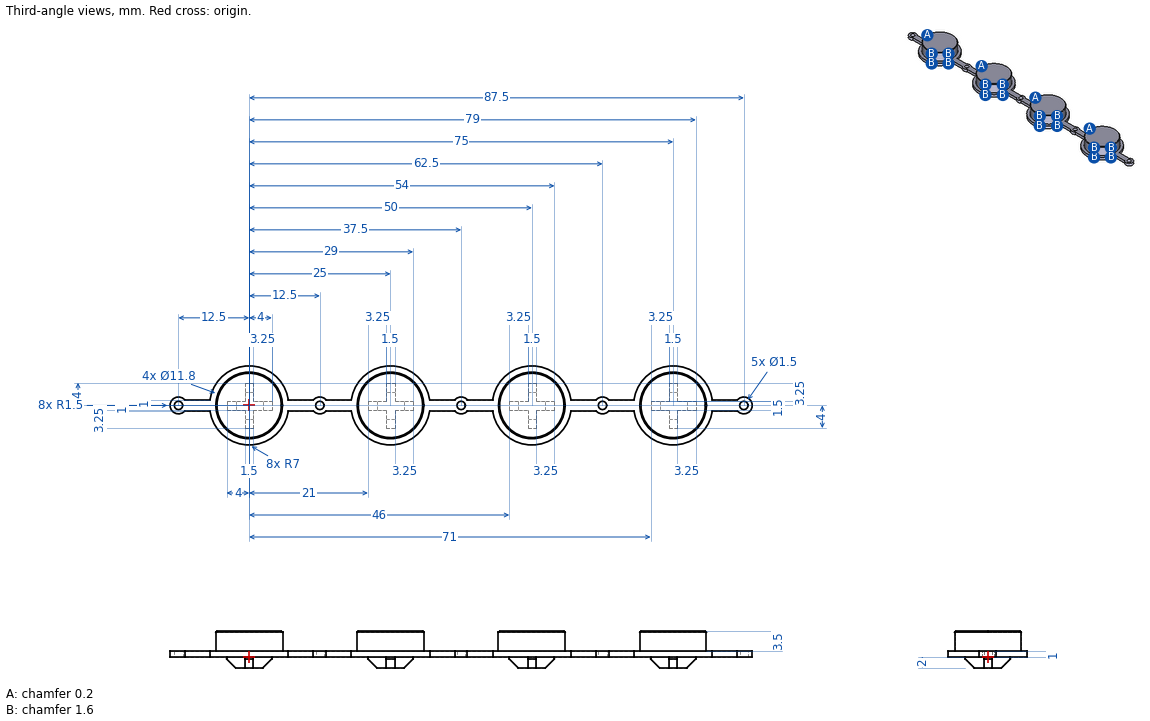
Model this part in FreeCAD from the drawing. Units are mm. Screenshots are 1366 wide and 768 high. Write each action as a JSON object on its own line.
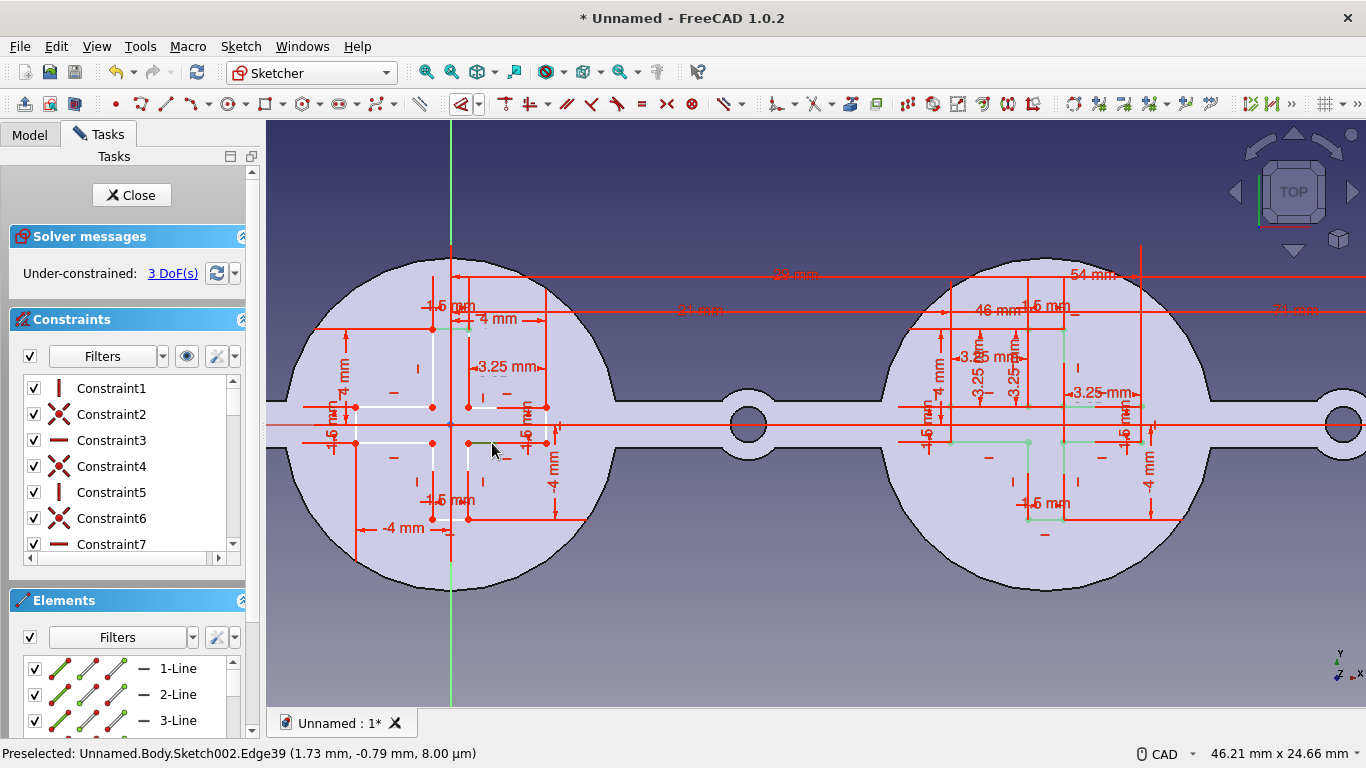
{"action": "key", "text": "l"}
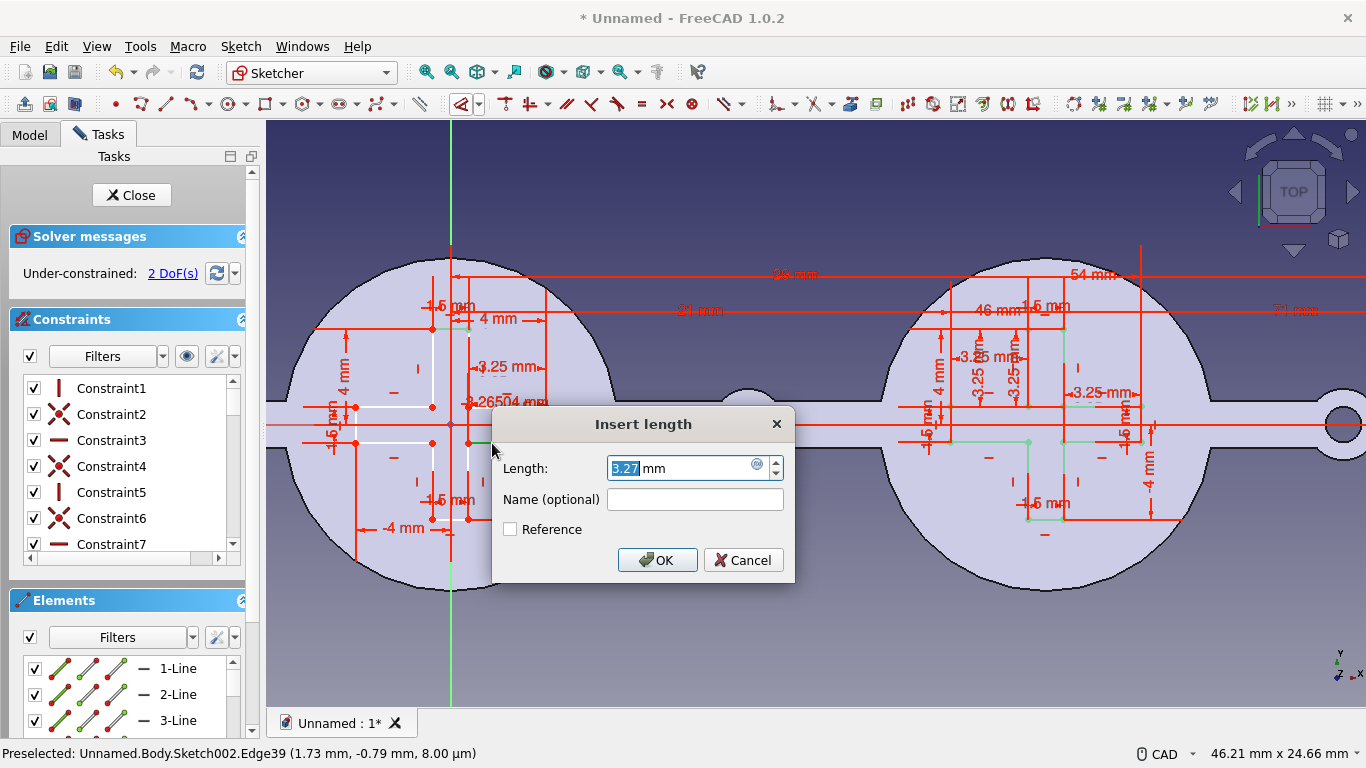
{"action": "type", "text": "3.25"}
{"action": "key", "text": "Return"}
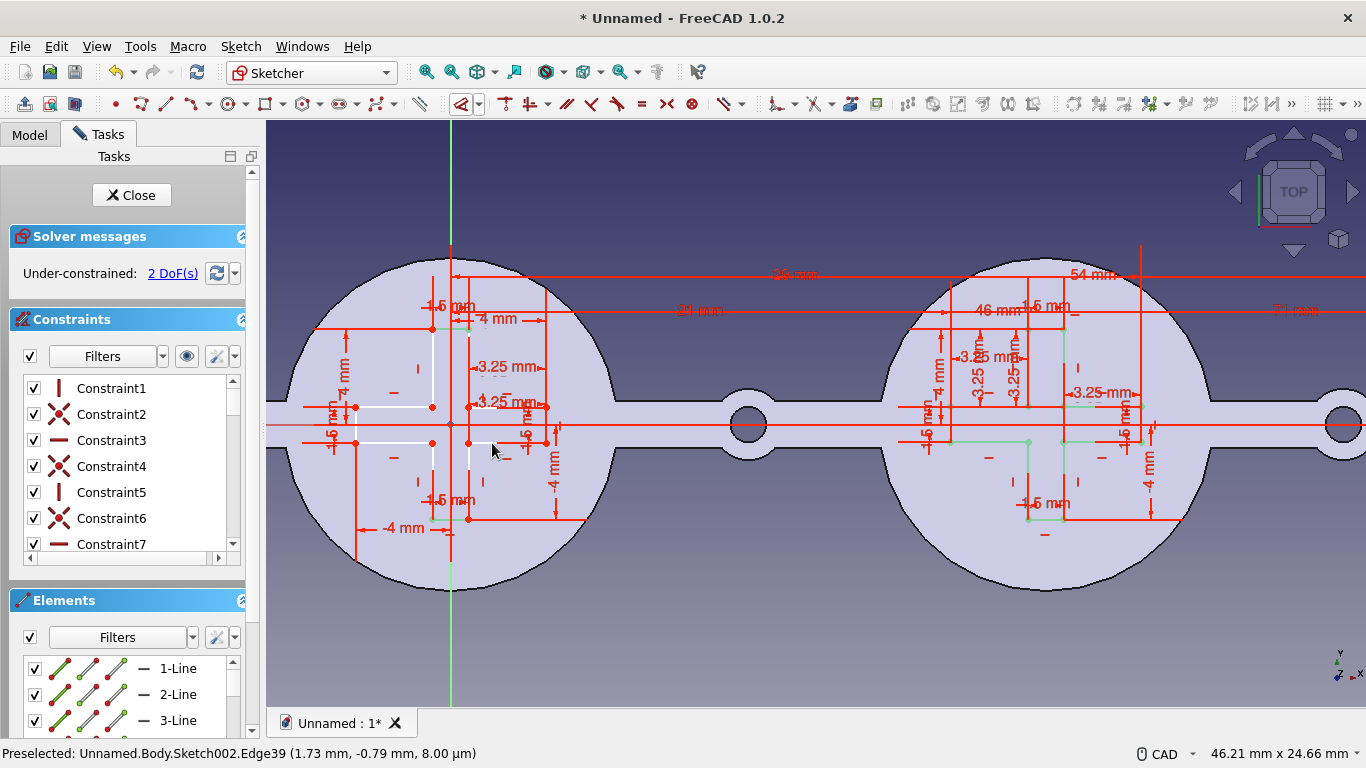
{"action": "left_click", "coordinate": [469, 466]}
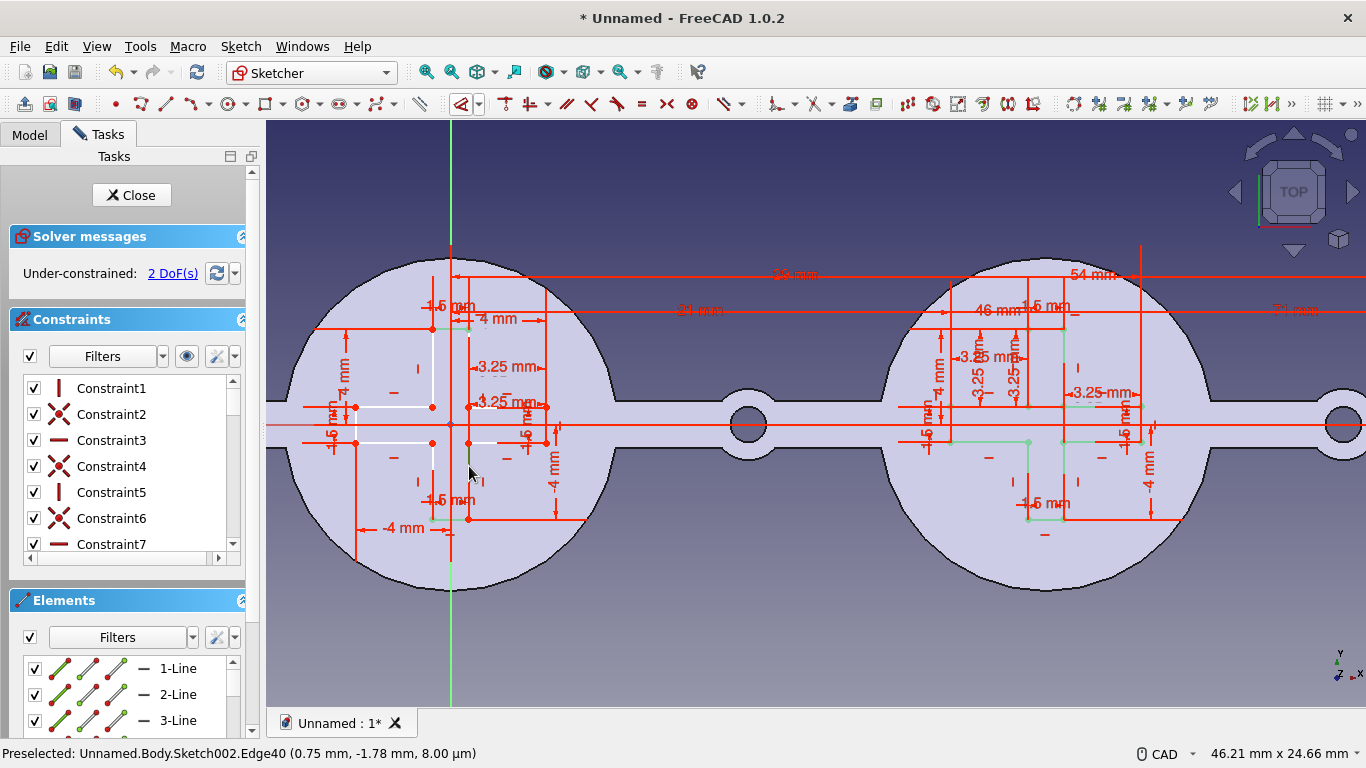
{"action": "key", "text": "i"}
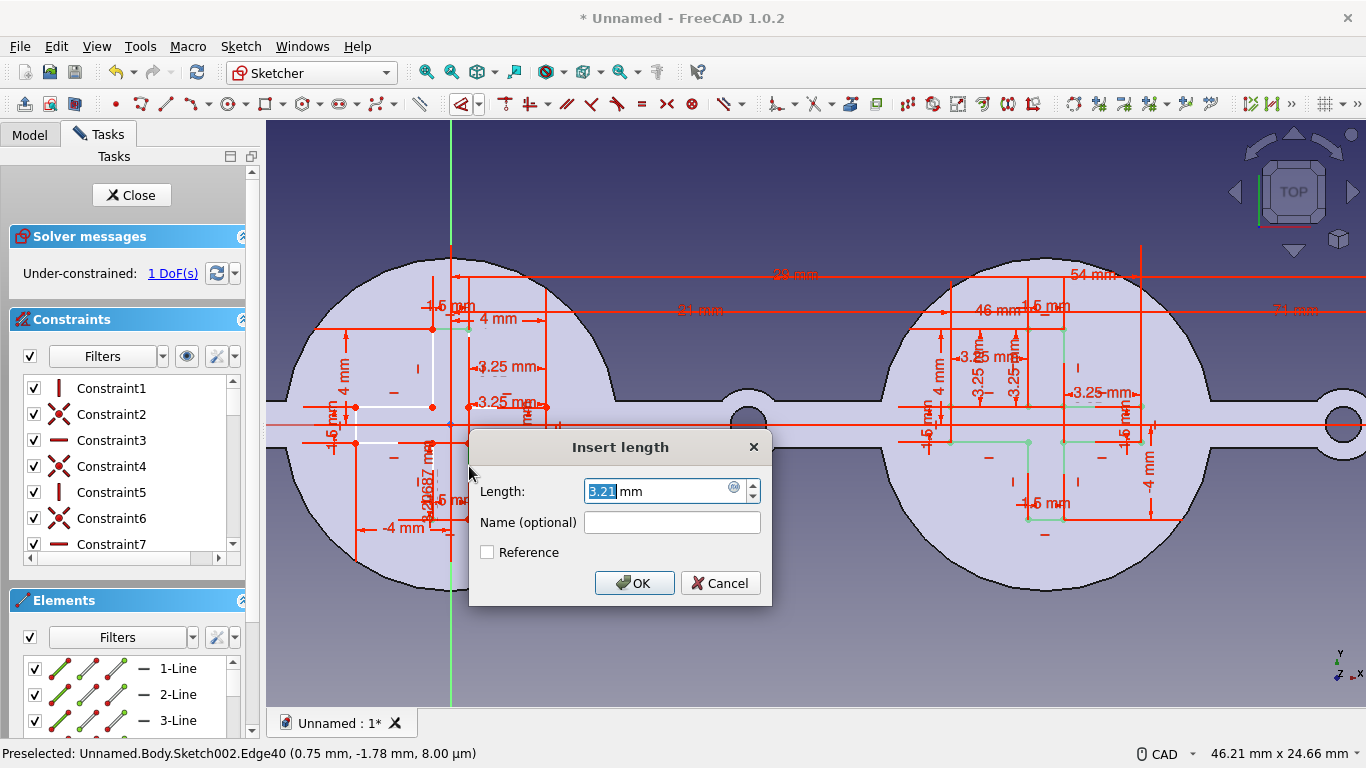
{"action": "type", "text": "3.25"}
{"action": "key", "text": "Return"}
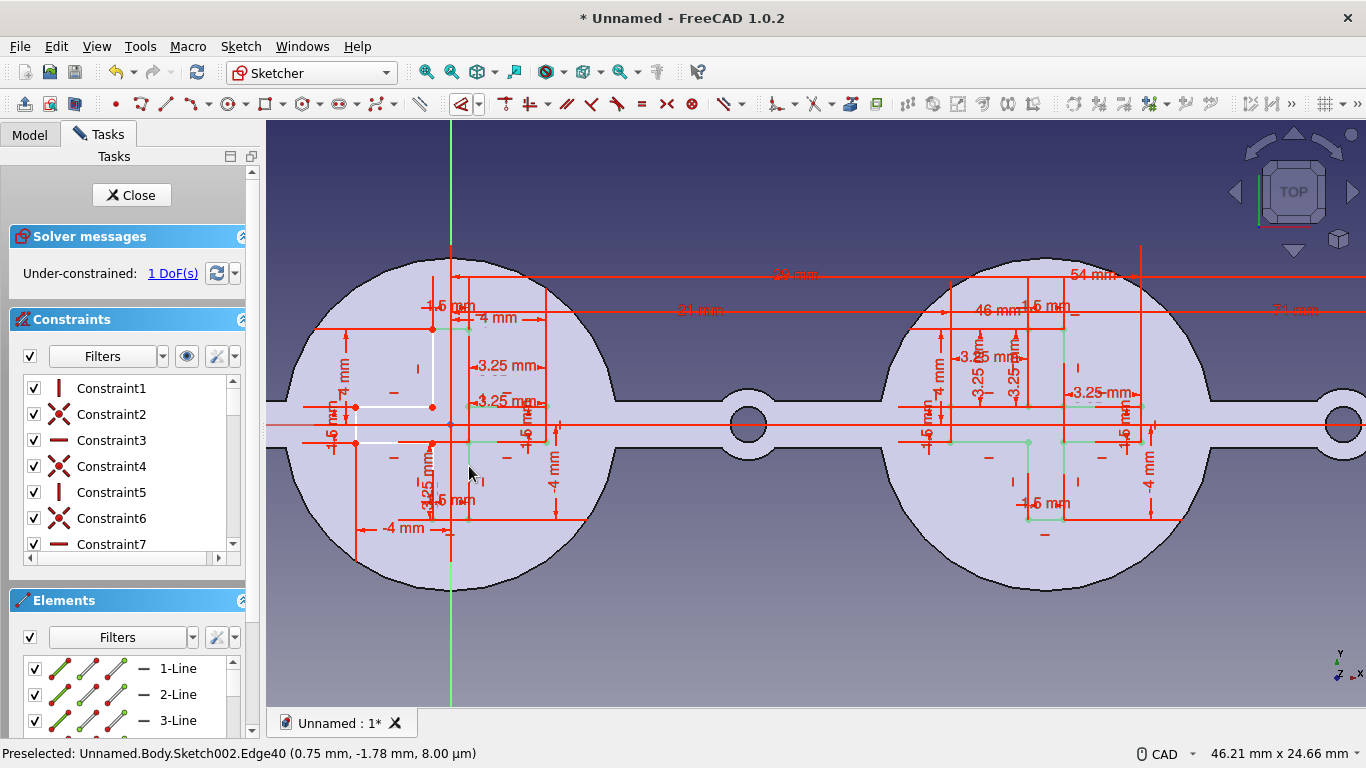
{"action": "scroll", "coordinate": [433, 497], "scroll_direction": "up", "scroll_amount": 4}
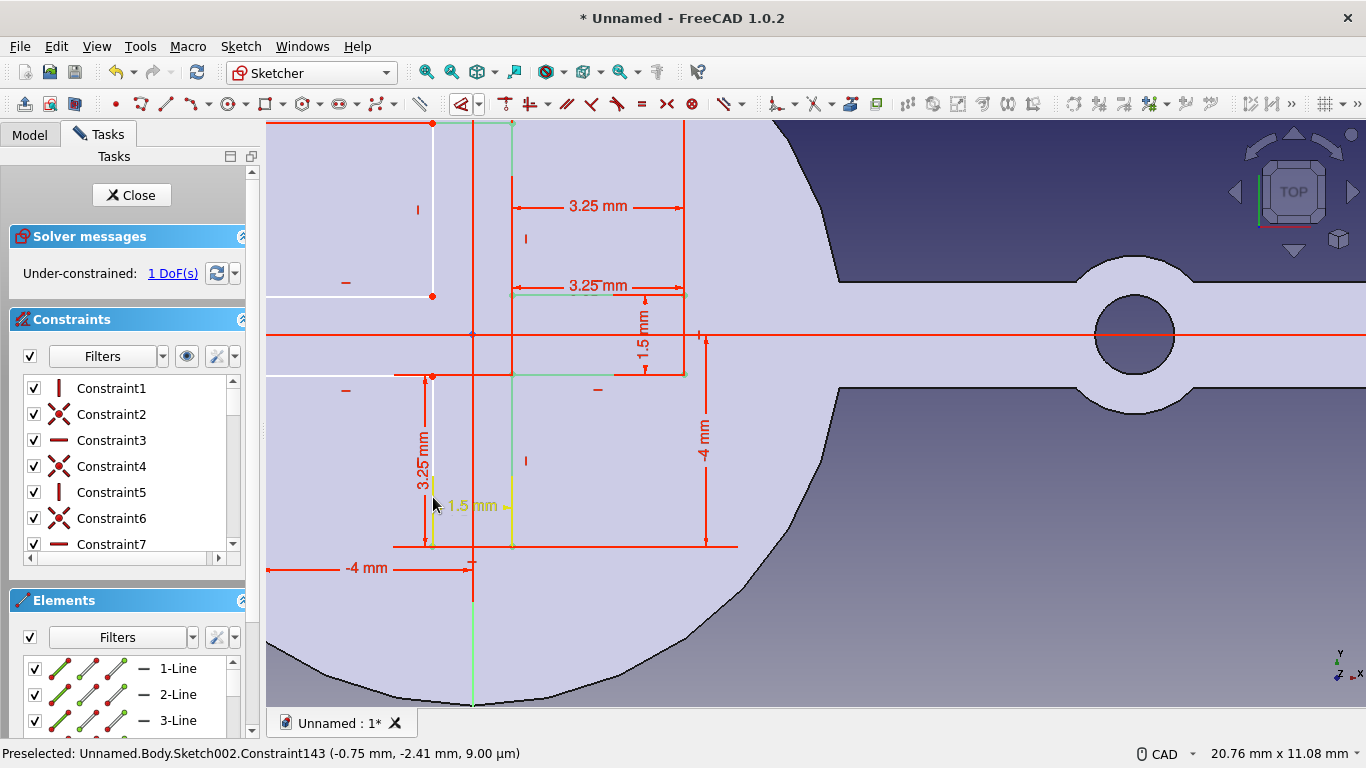
{"action": "left_click", "coordinate": [433, 496]}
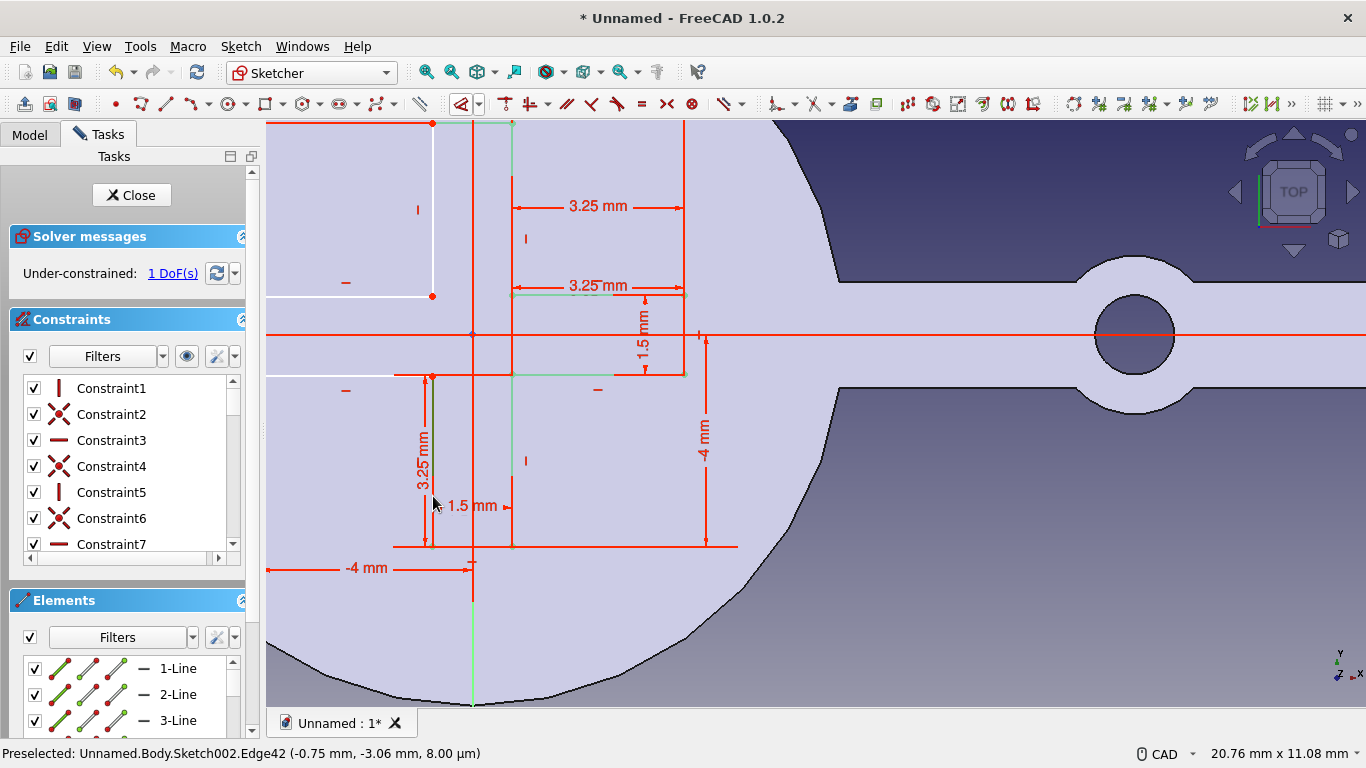
{"action": "key", "text": "i"}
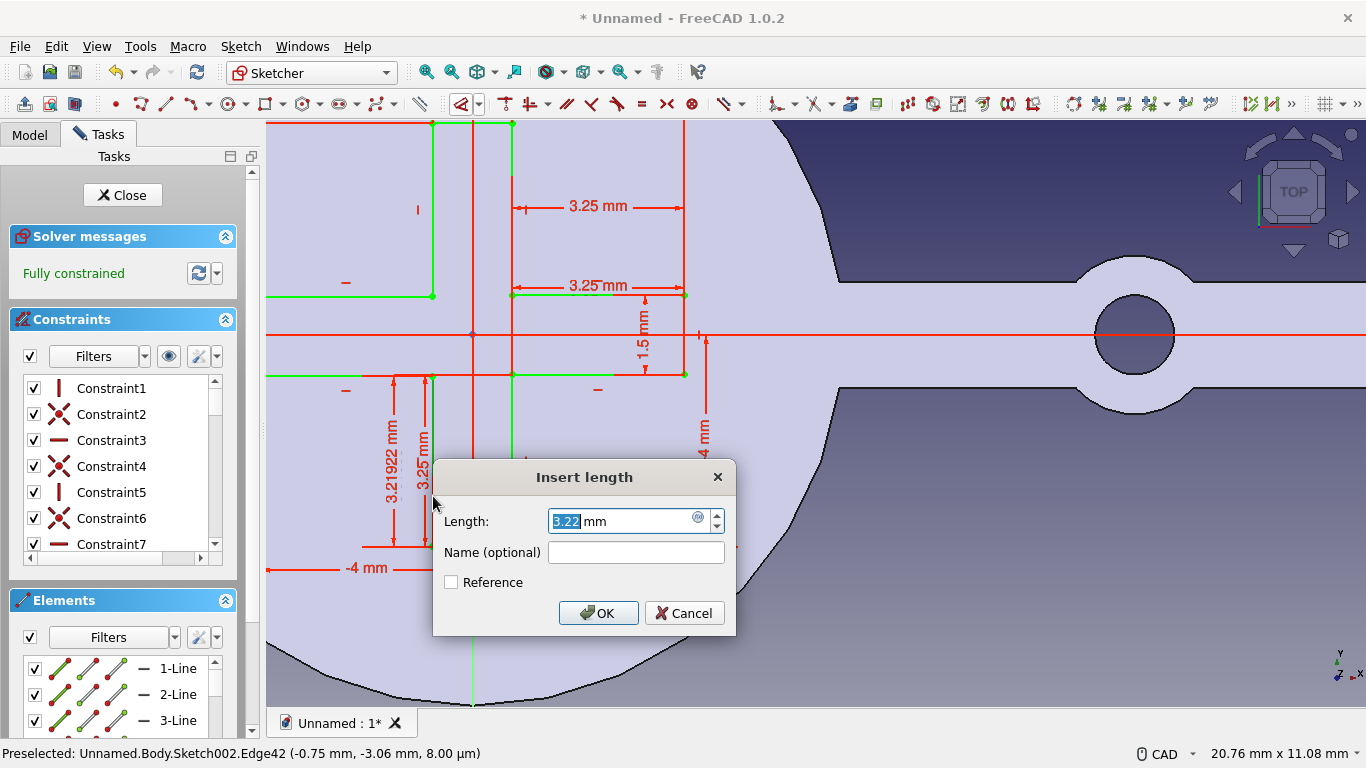
{"action": "type", "text": "3.25"}
{"action": "key", "text": "Return"}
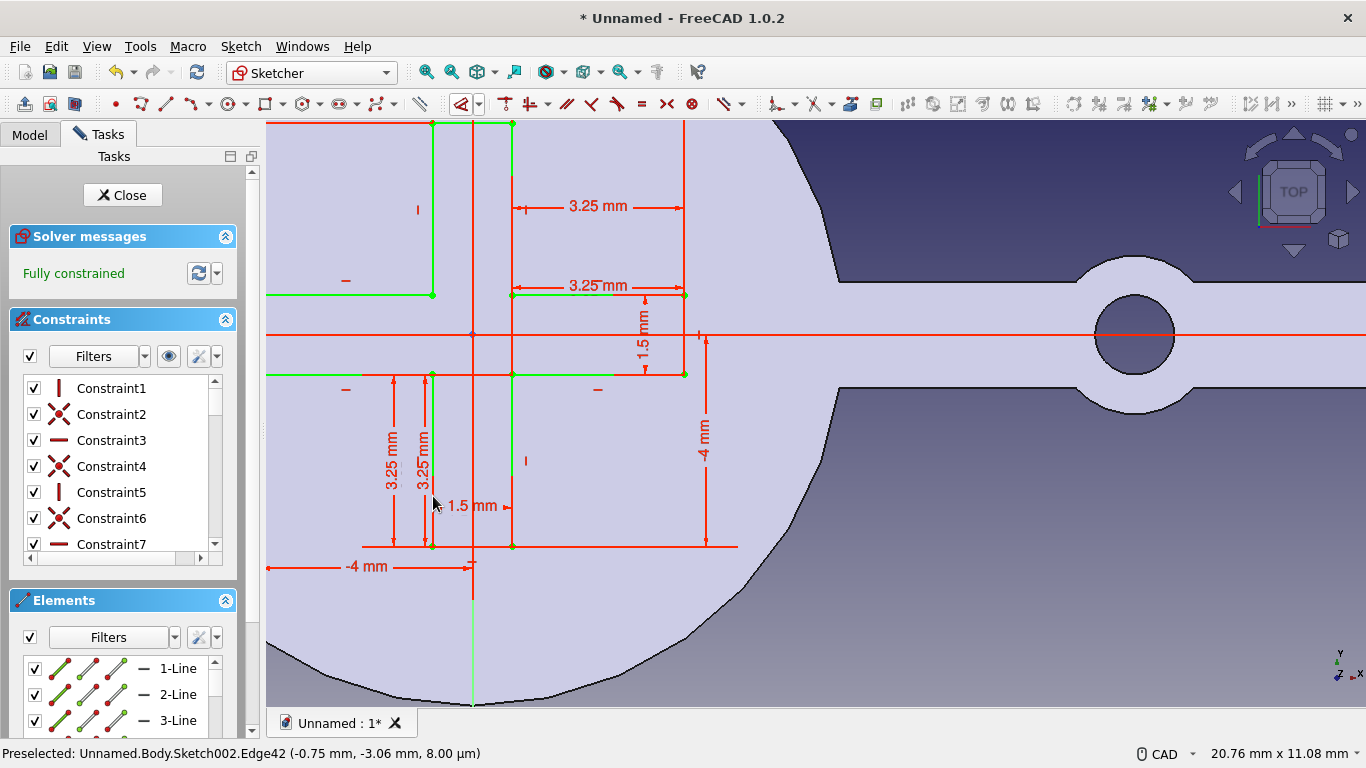
{"action": "left_click", "coordinate": [123, 195]}